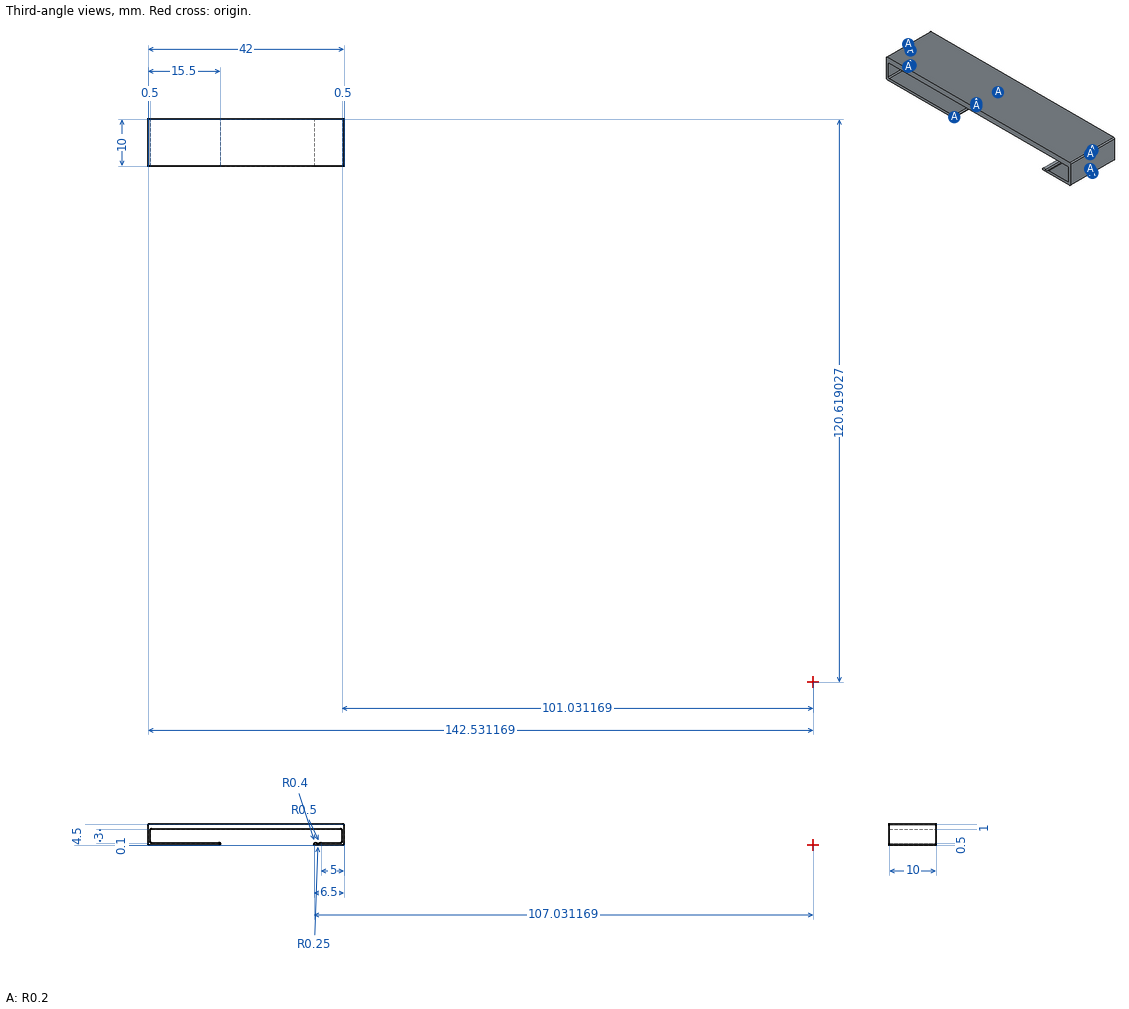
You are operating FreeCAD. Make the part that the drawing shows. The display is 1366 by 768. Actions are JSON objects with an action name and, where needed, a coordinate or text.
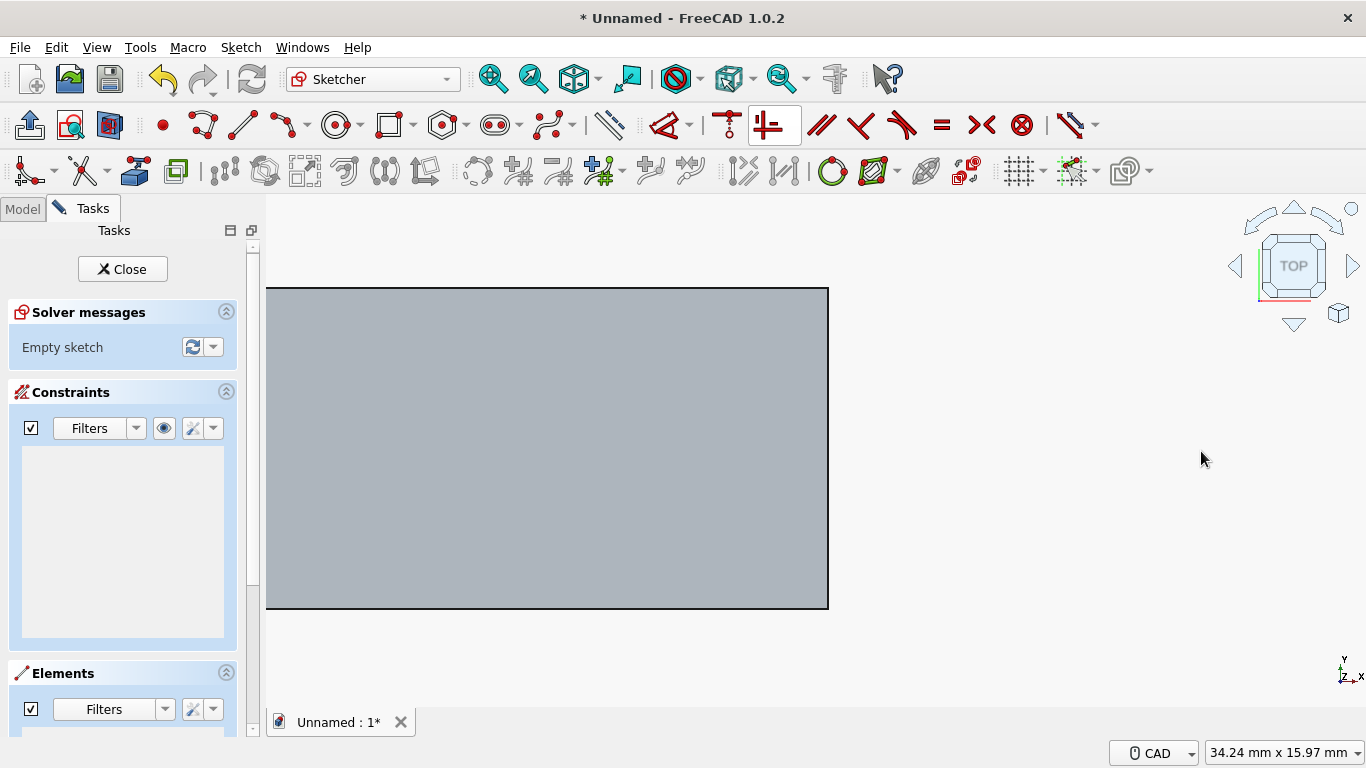
{"action": "left_click", "coordinate": [390, 126]}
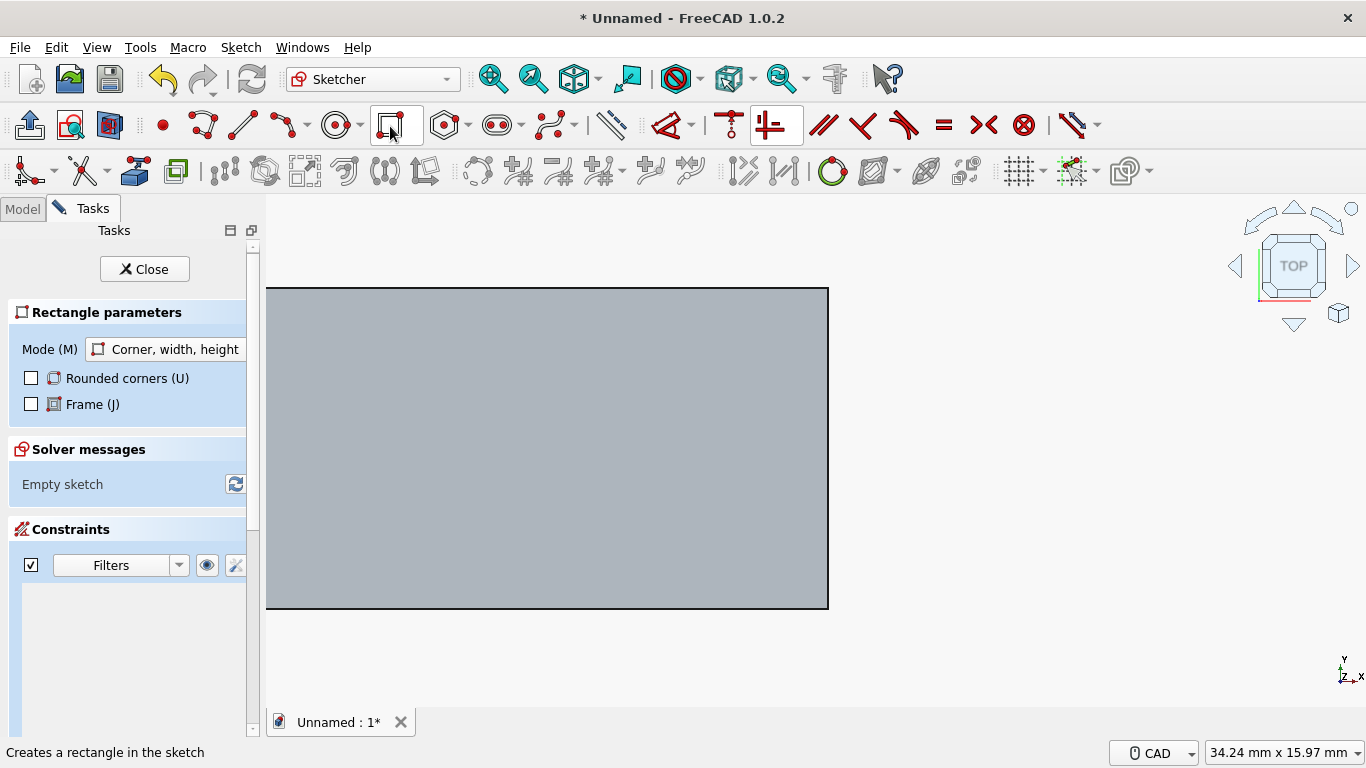
{"action": "left_click", "coordinate": [812, 288]}
{"action": "left_click", "coordinate": [828, 609]}
{"action": "key", "text": "Escape"}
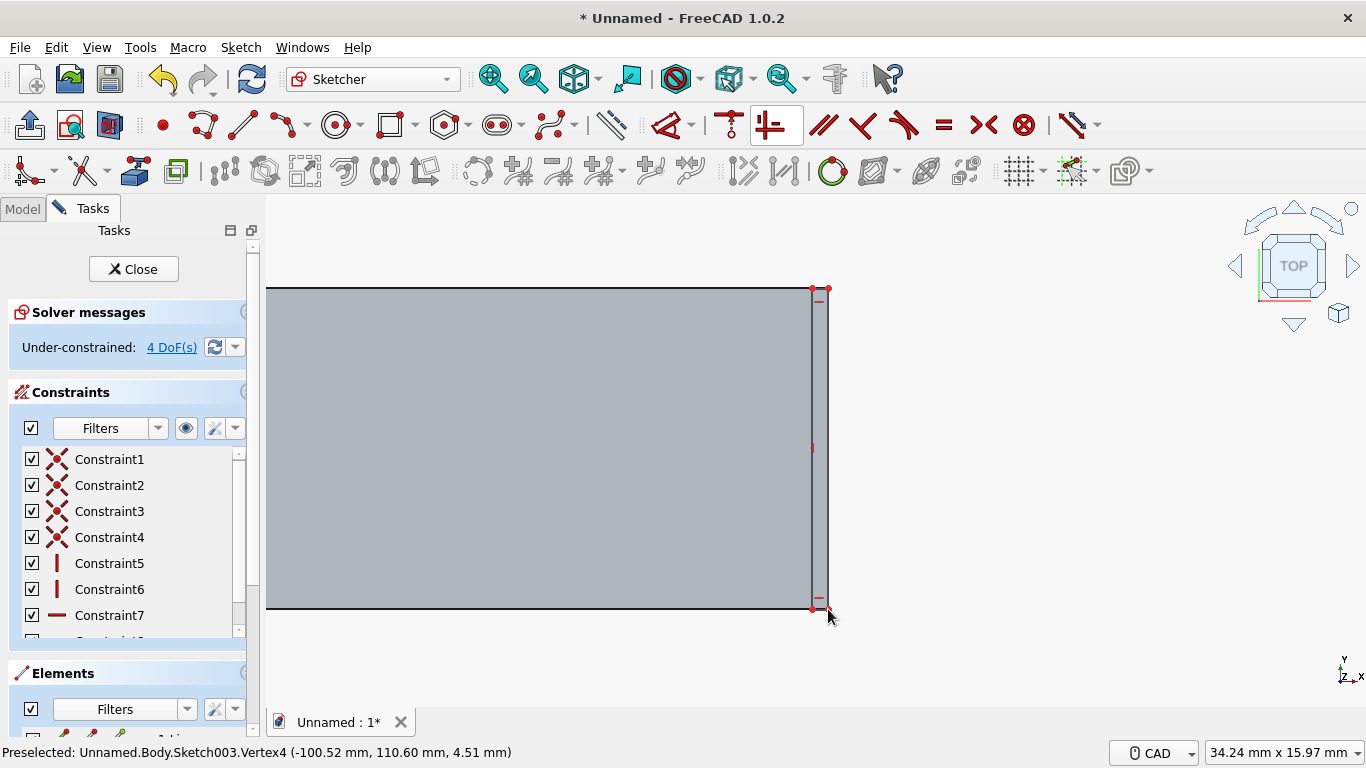
{"action": "left_click", "coordinate": [666, 126]}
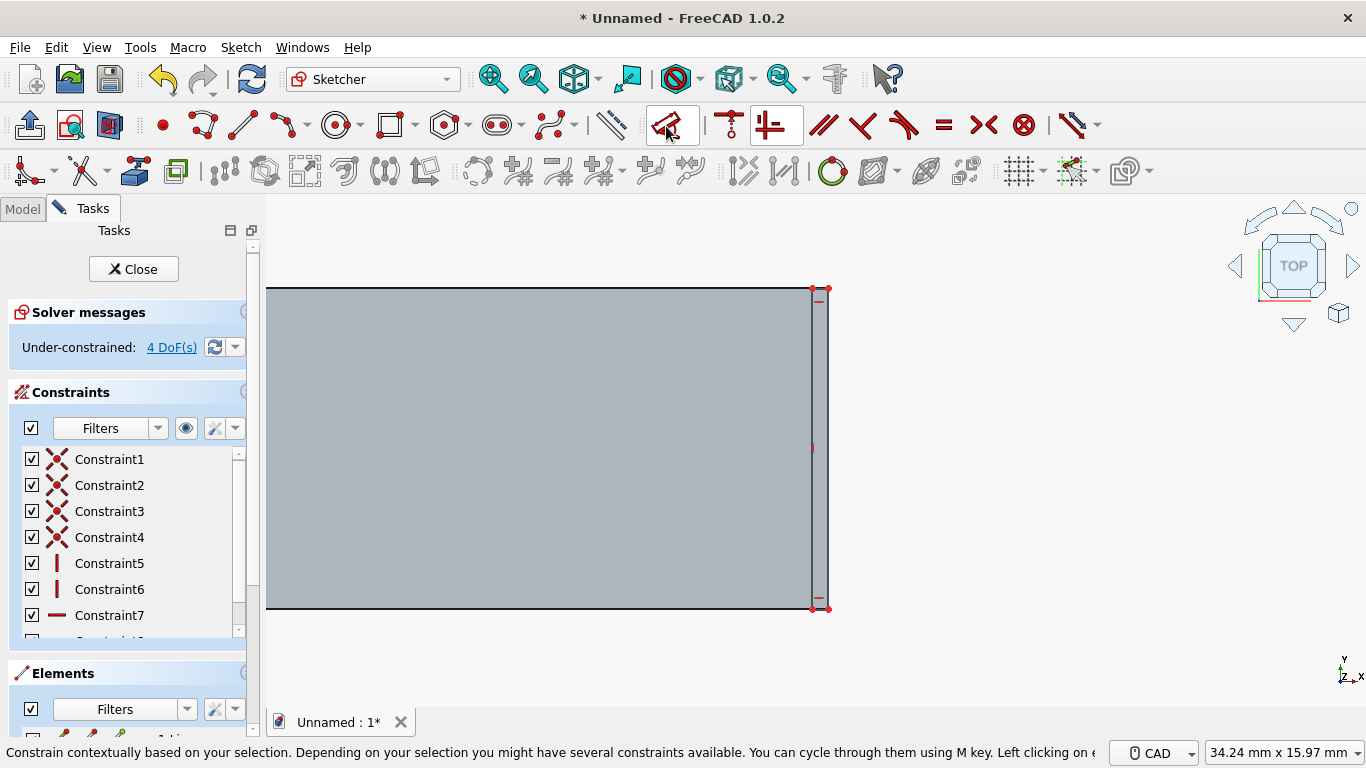
{"action": "left_click", "coordinate": [812, 385]}
{"action": "left_click", "coordinate": [778, 450]}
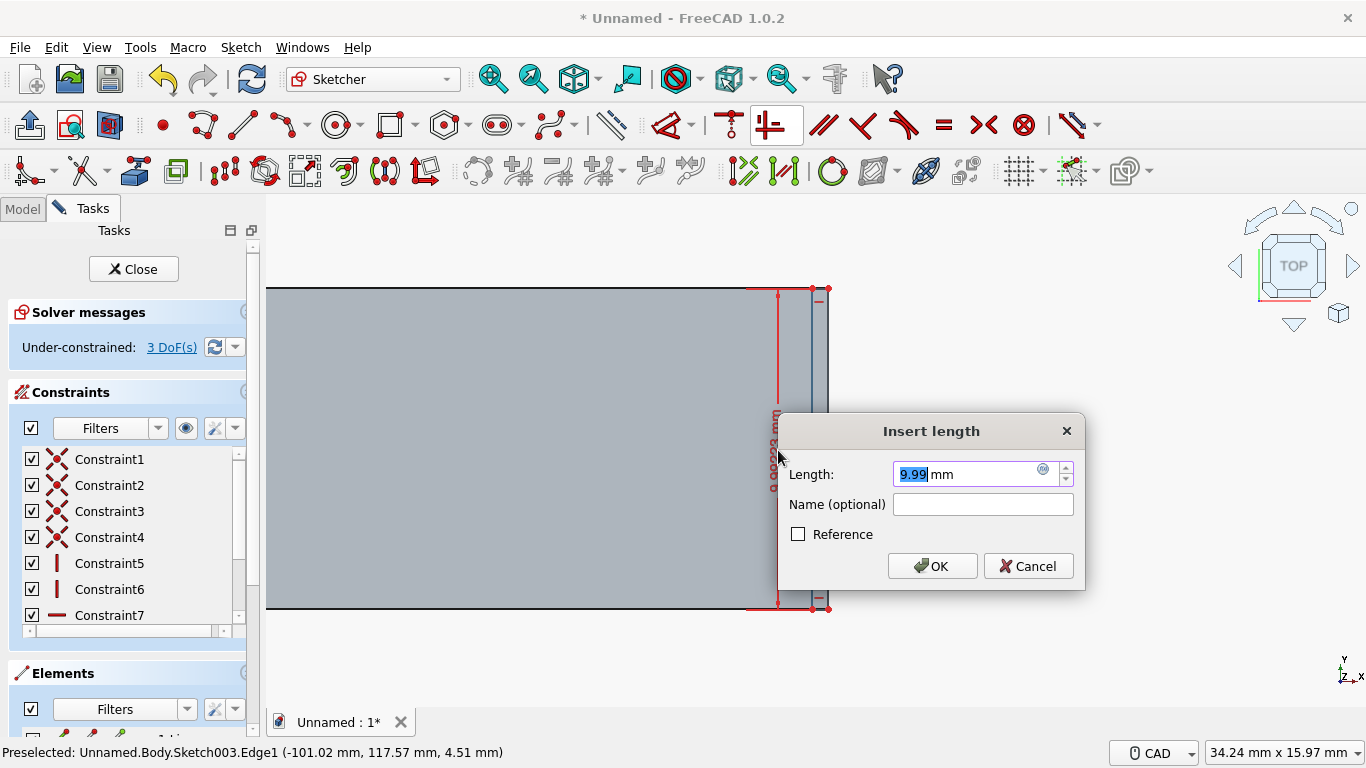
{"action": "type", "text": "10"}
{"action": "key", "text": "Return"}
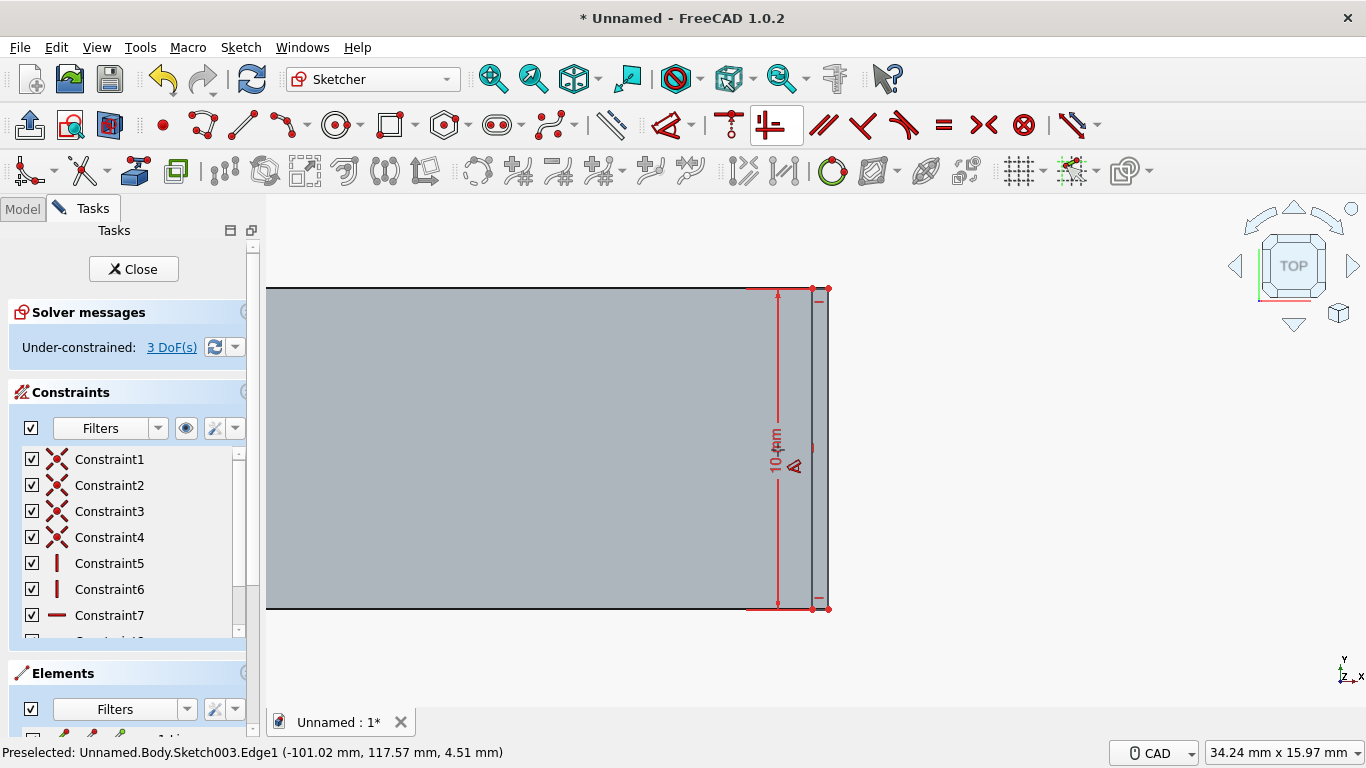
{"action": "scroll", "coordinate": [820, 610], "scroll_direction": "up", "scroll_amount": 5}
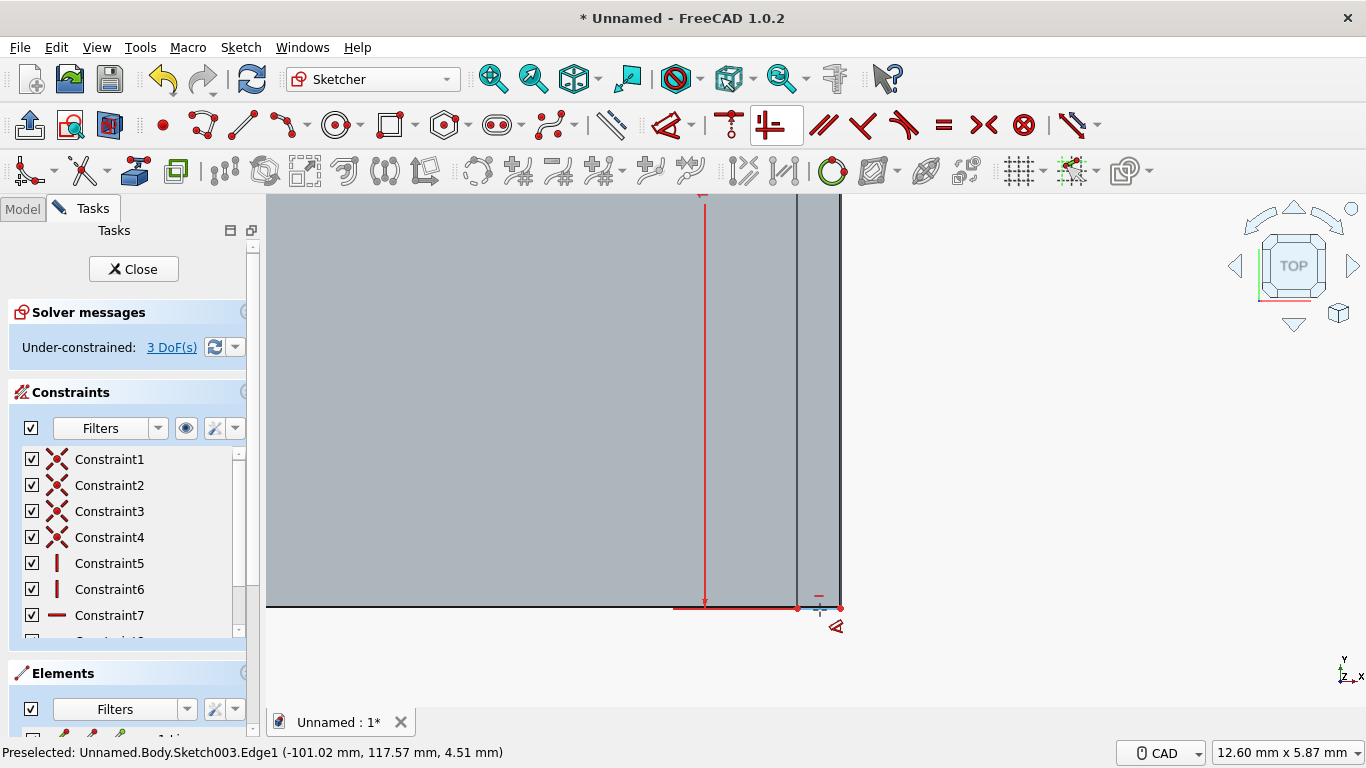
{"action": "left_click", "coordinate": [819, 609]}
{"action": "left_click", "coordinate": [819, 643]}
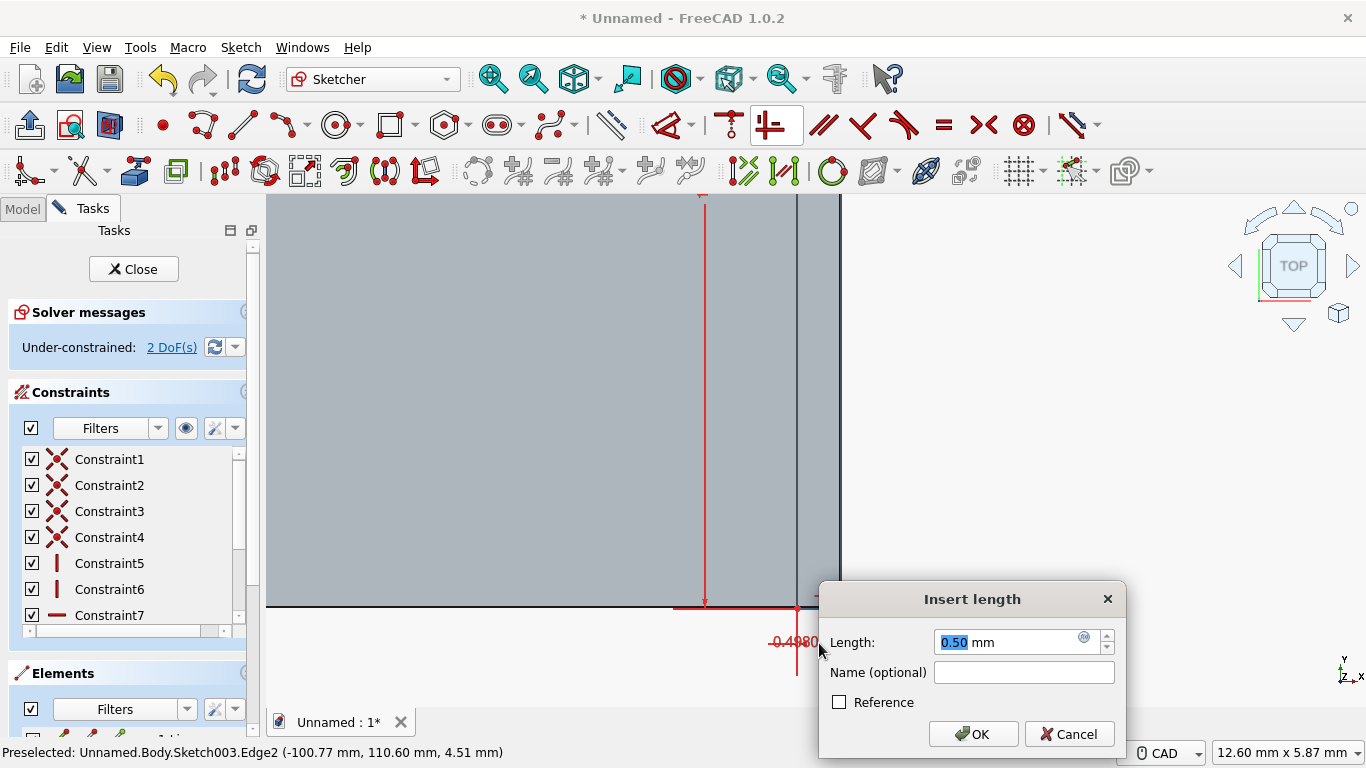
{"action": "type", "text": "0.5"}
{"action": "key", "text": "Return"}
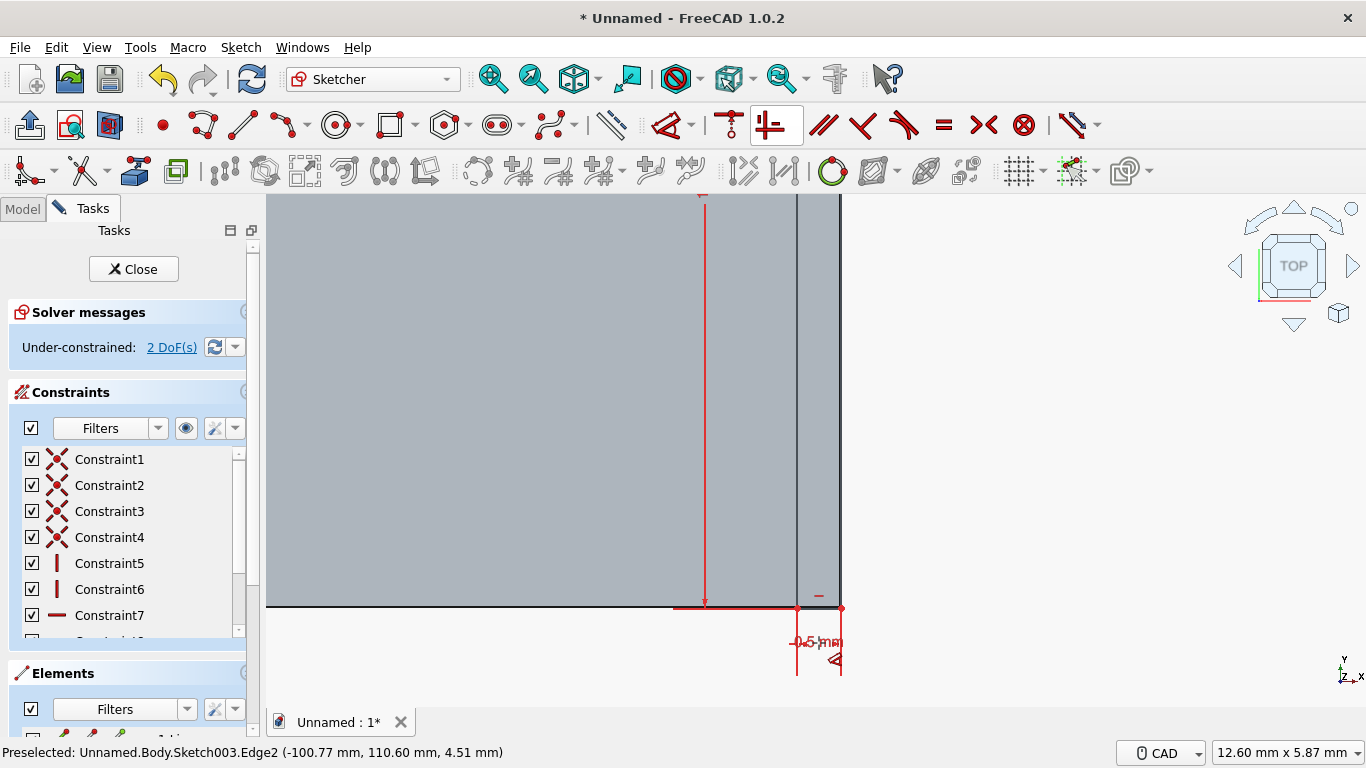
{"action": "scroll", "coordinate": [706, 614], "scroll_direction": "down", "scroll_amount": 5}